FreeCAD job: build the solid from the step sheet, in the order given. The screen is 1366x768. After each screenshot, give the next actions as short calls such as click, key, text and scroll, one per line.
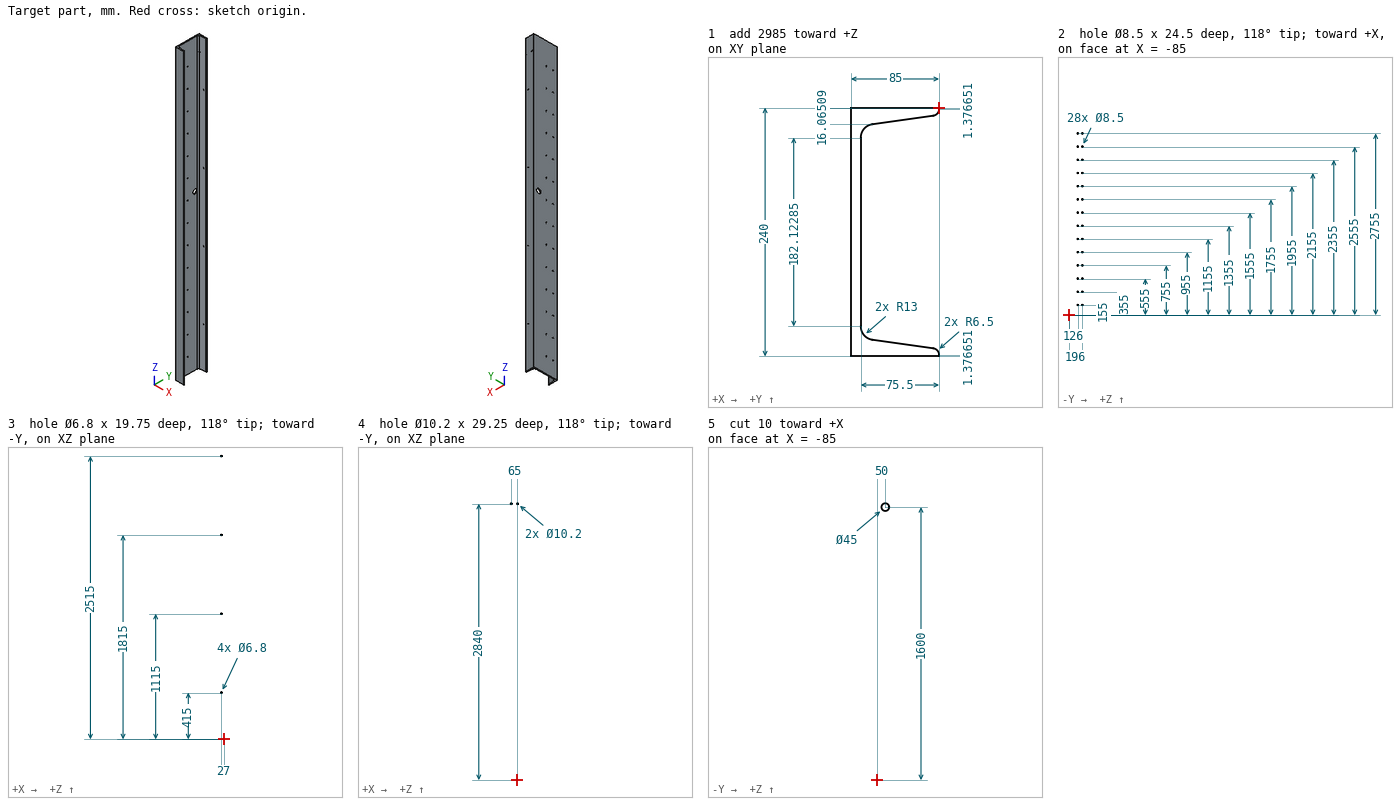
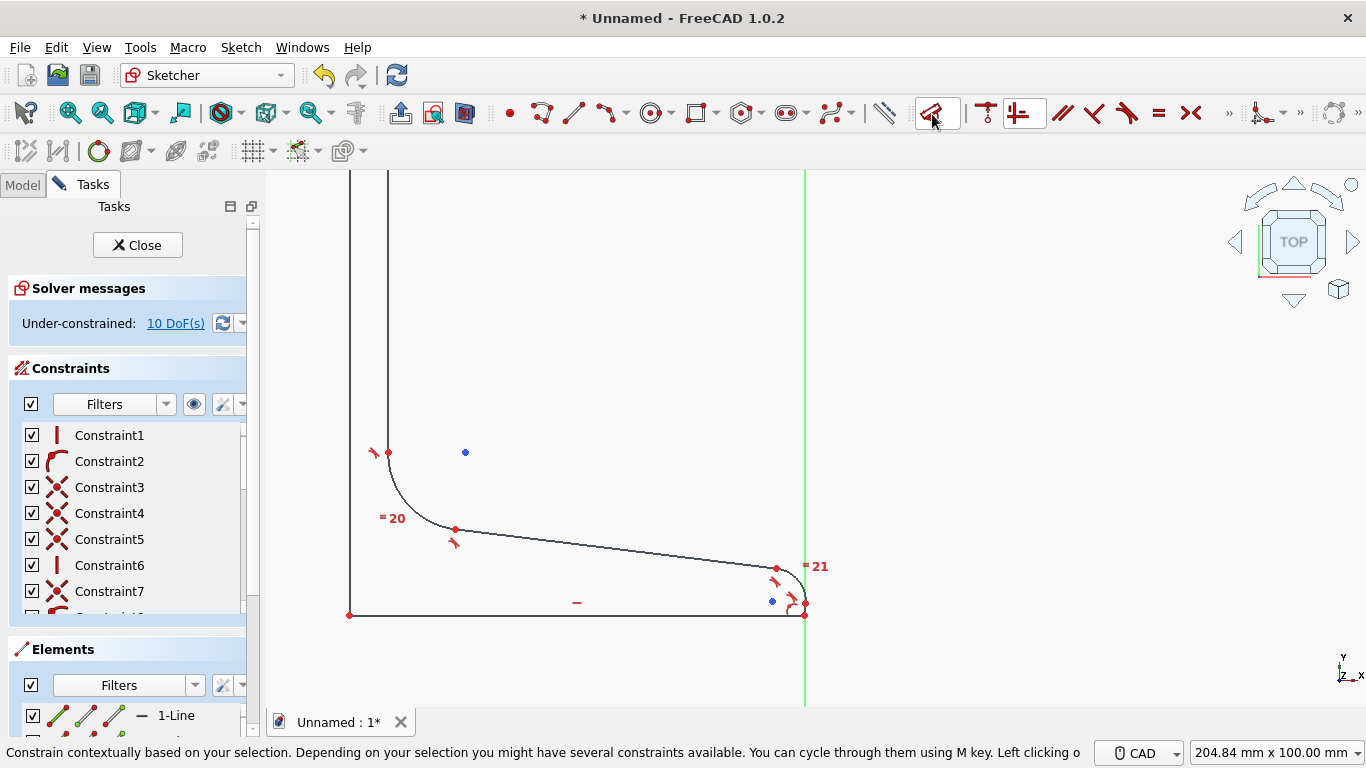
click(395, 485)
click(366, 498)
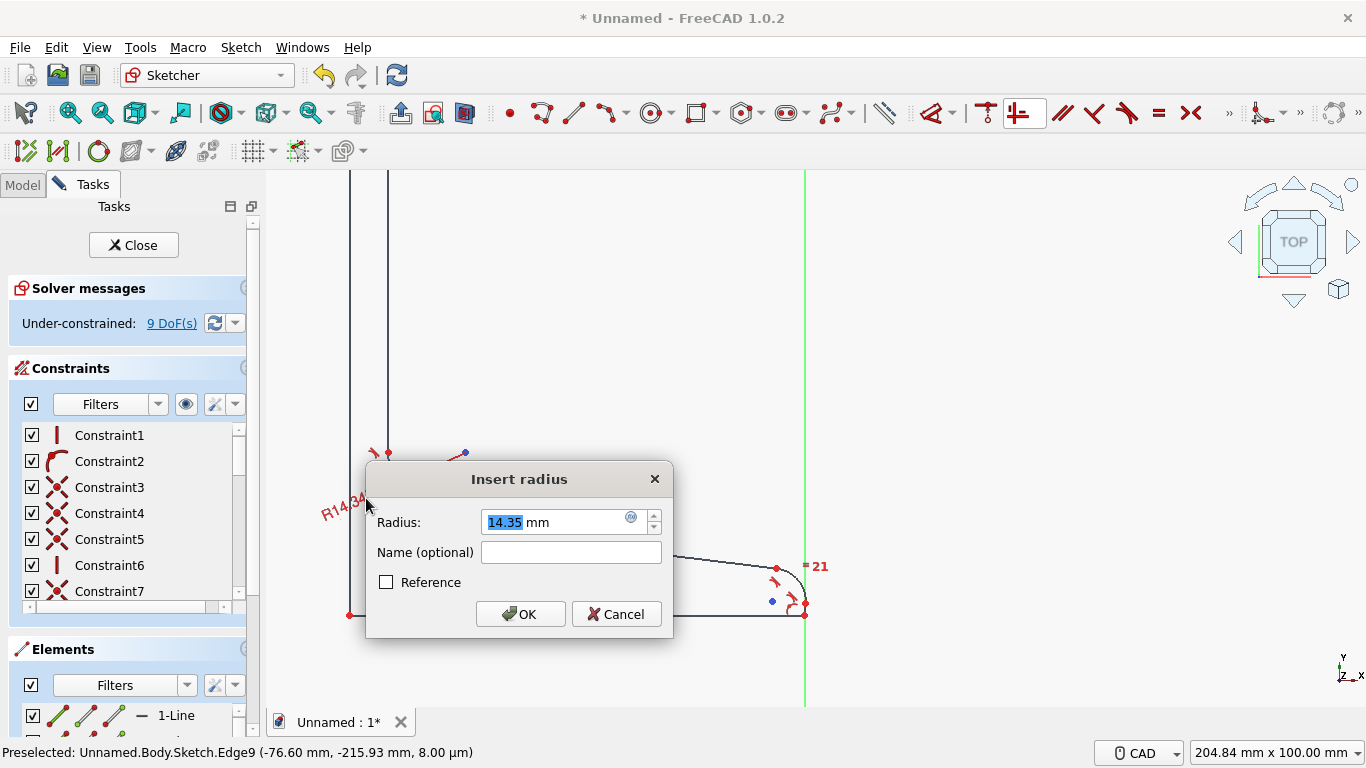
text(13)
key(Return)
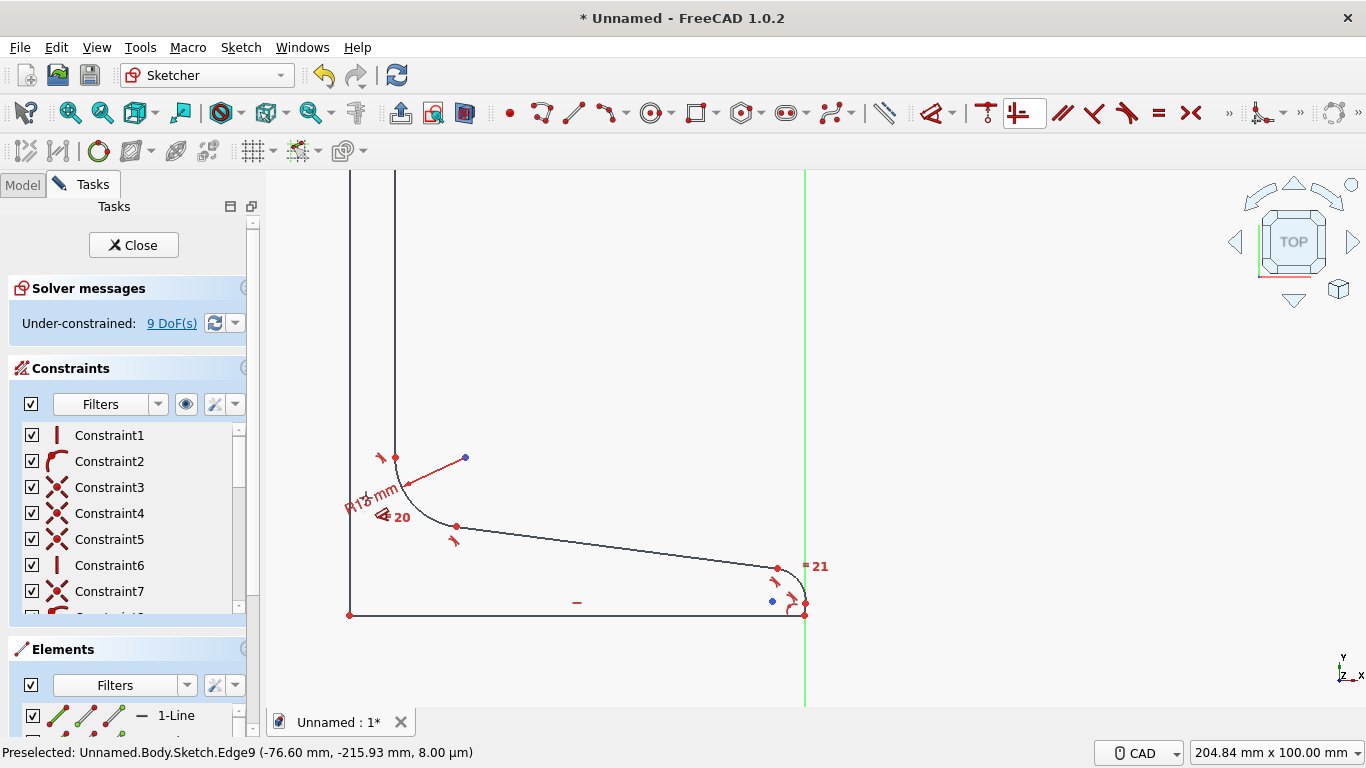
scroll(803, 593, down, 7)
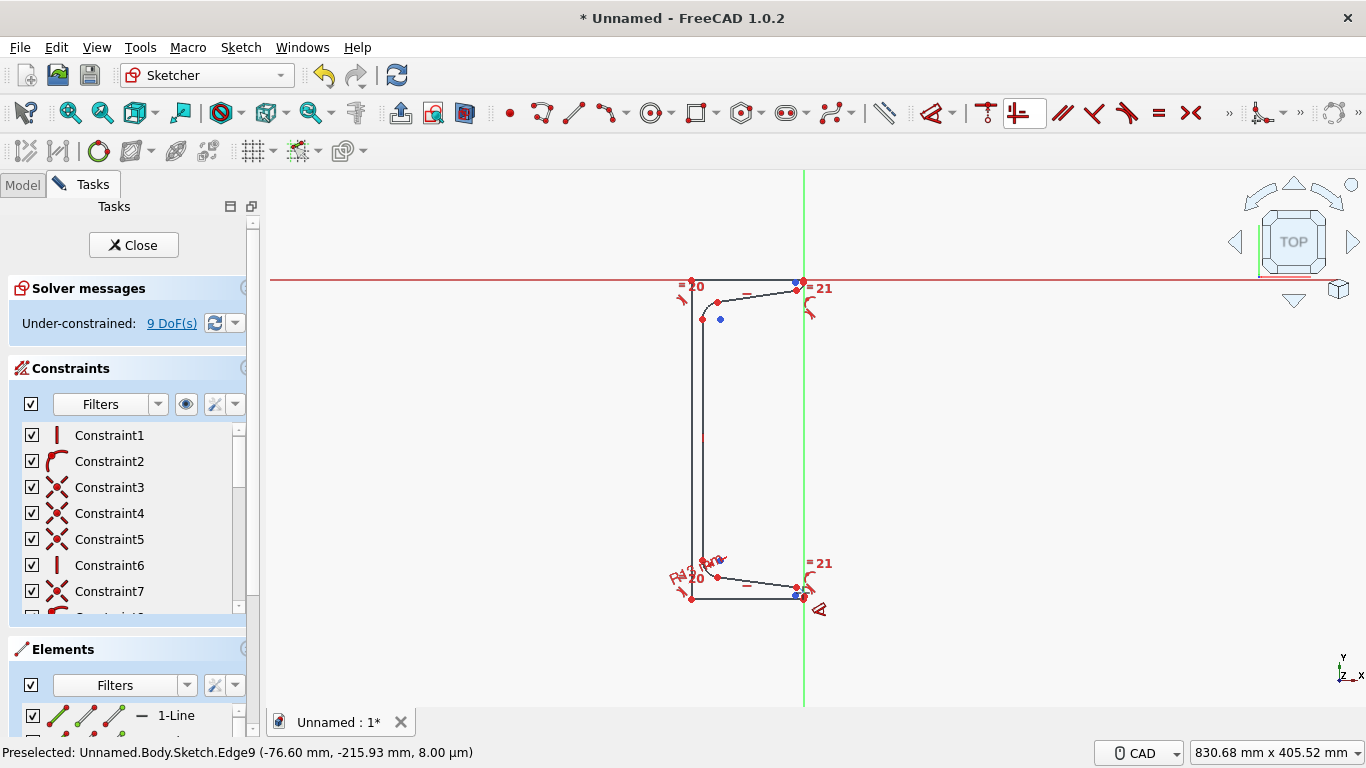
scroll(800, 289, up, 8)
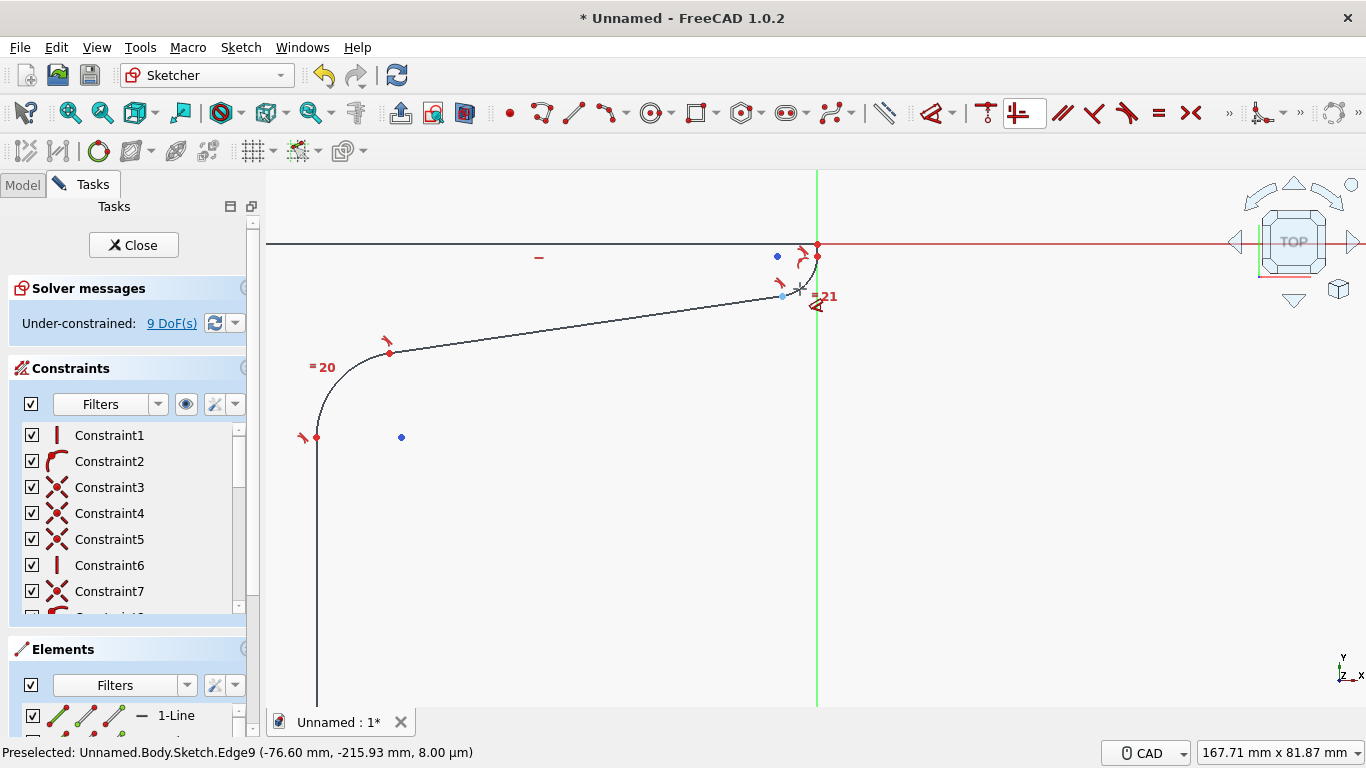
click(799, 290)
click(783, 328)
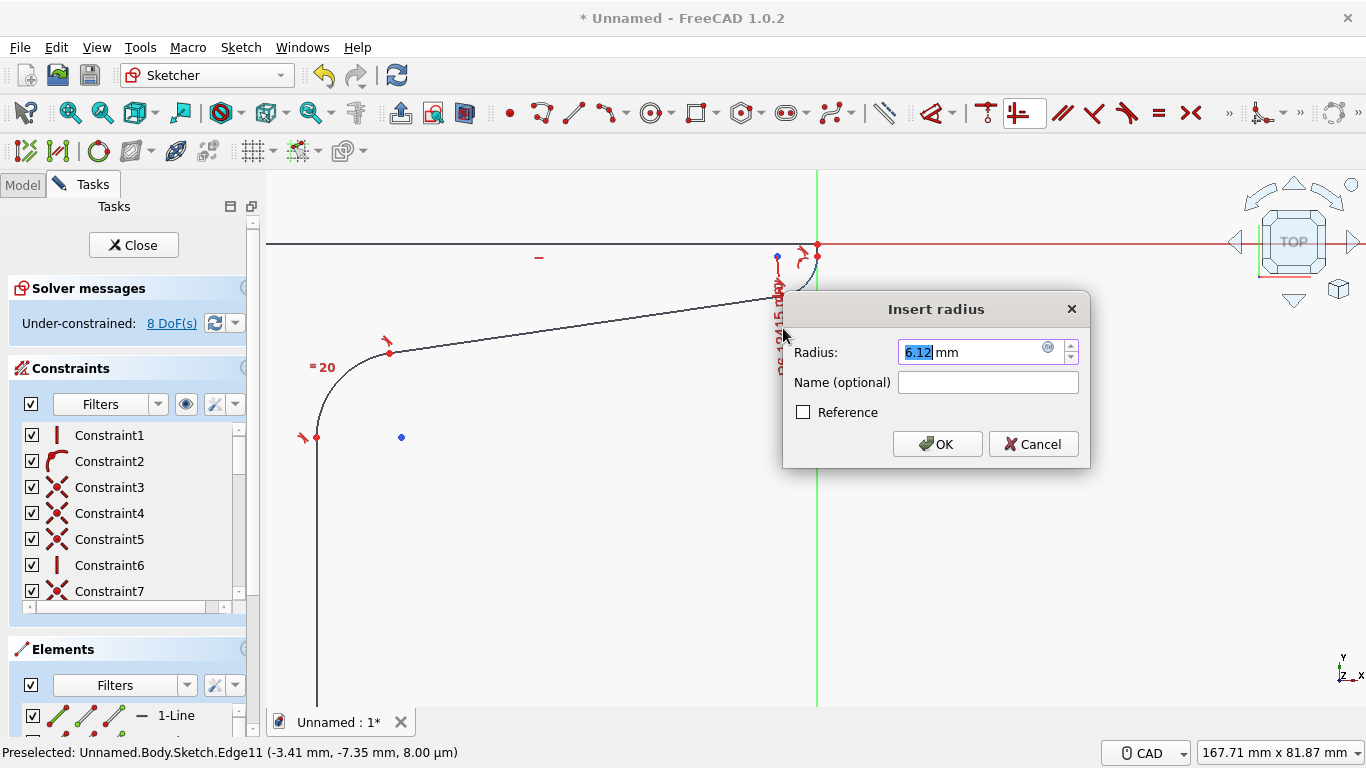
text(6.5)
key(Return)
key(Escape)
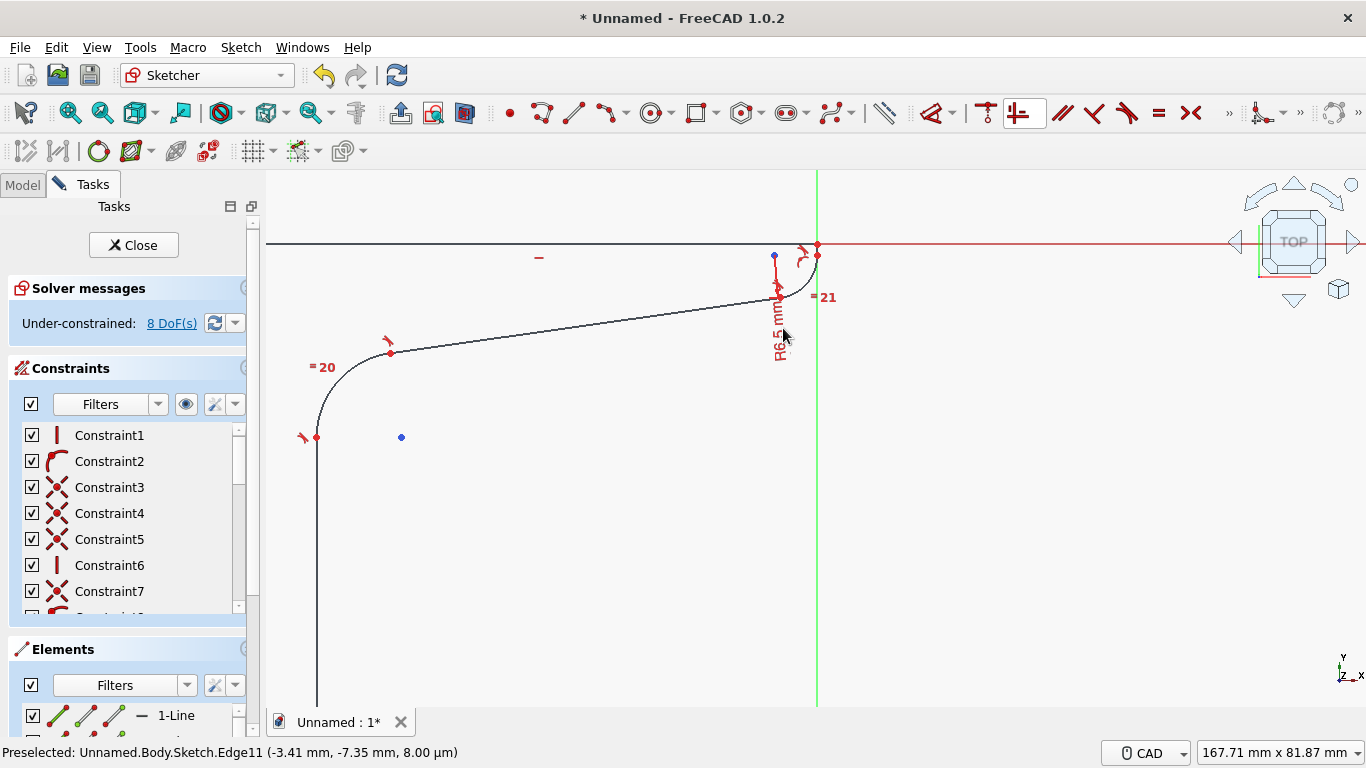
scroll(800, 289, down, 8)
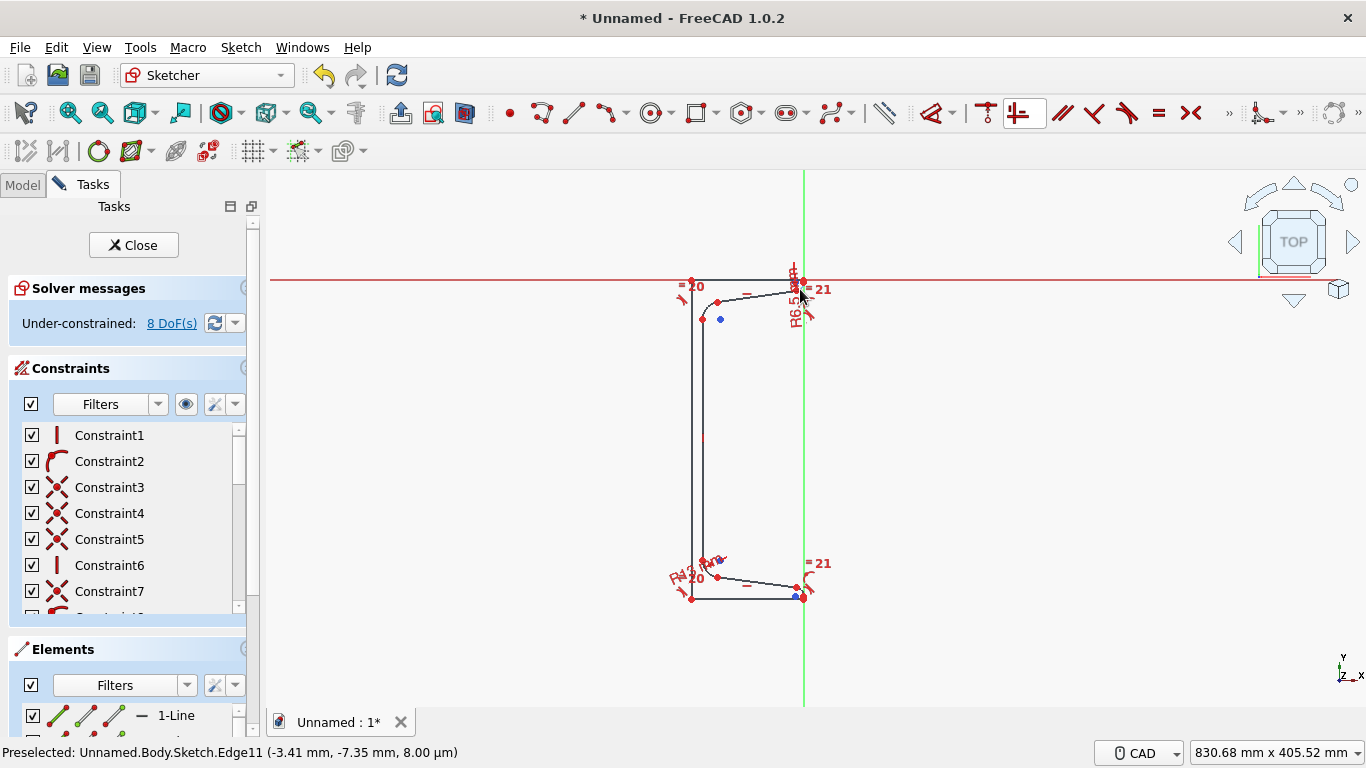
scroll(804, 596, up, 7)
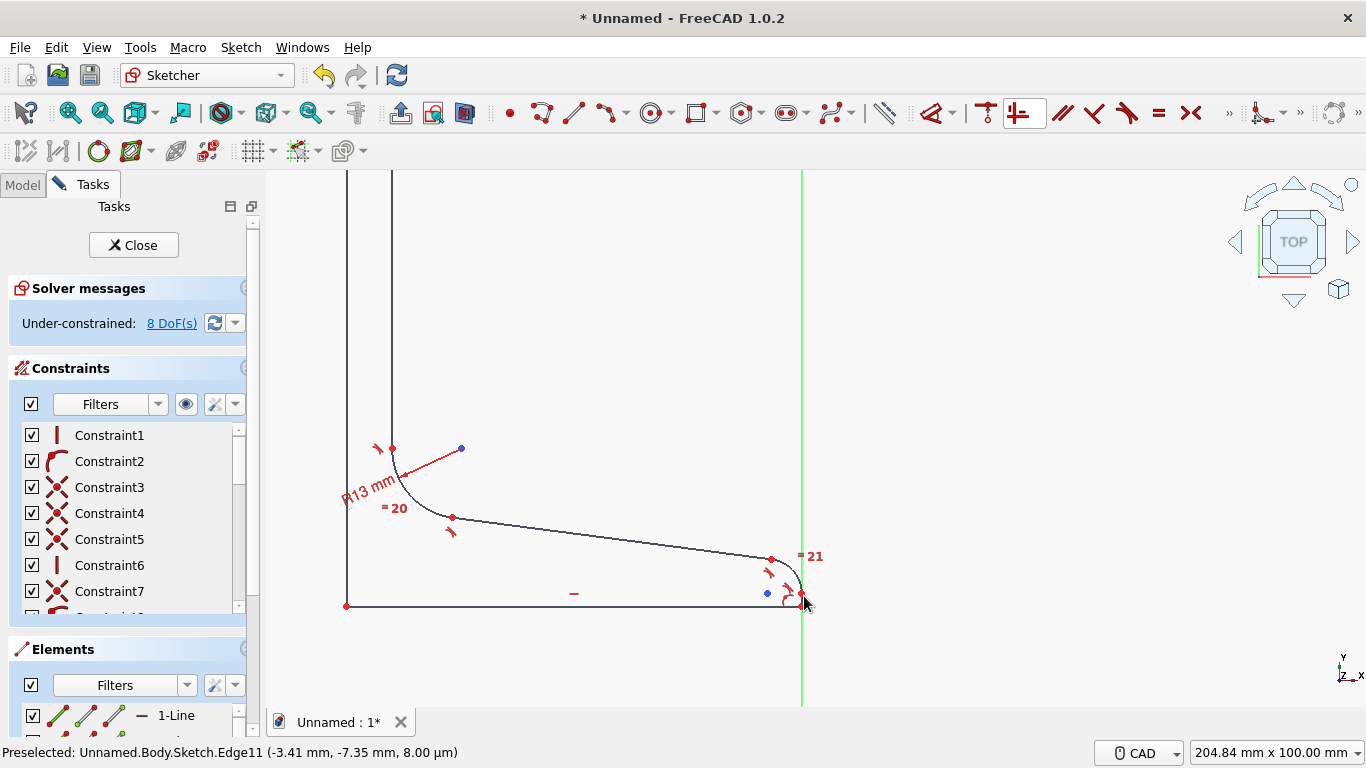
click(802, 594)